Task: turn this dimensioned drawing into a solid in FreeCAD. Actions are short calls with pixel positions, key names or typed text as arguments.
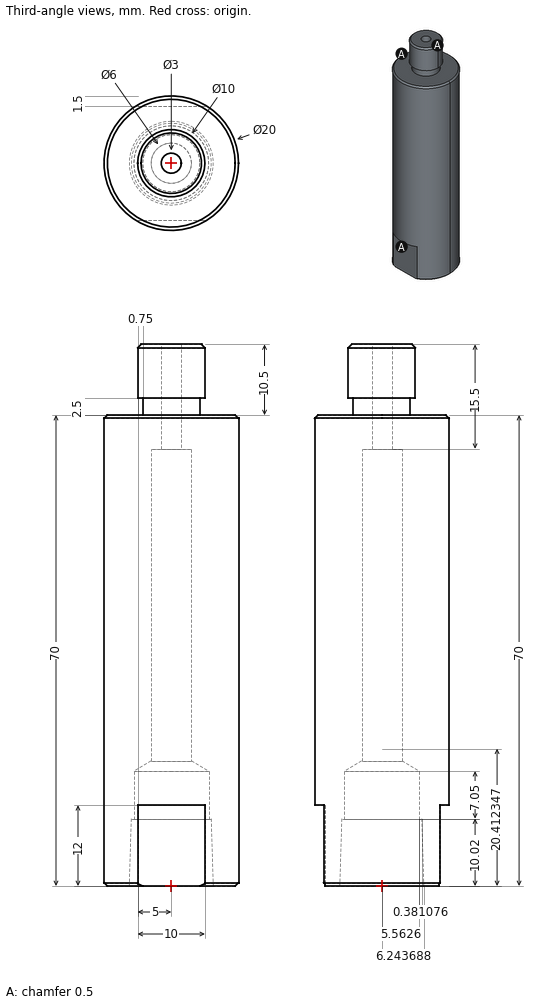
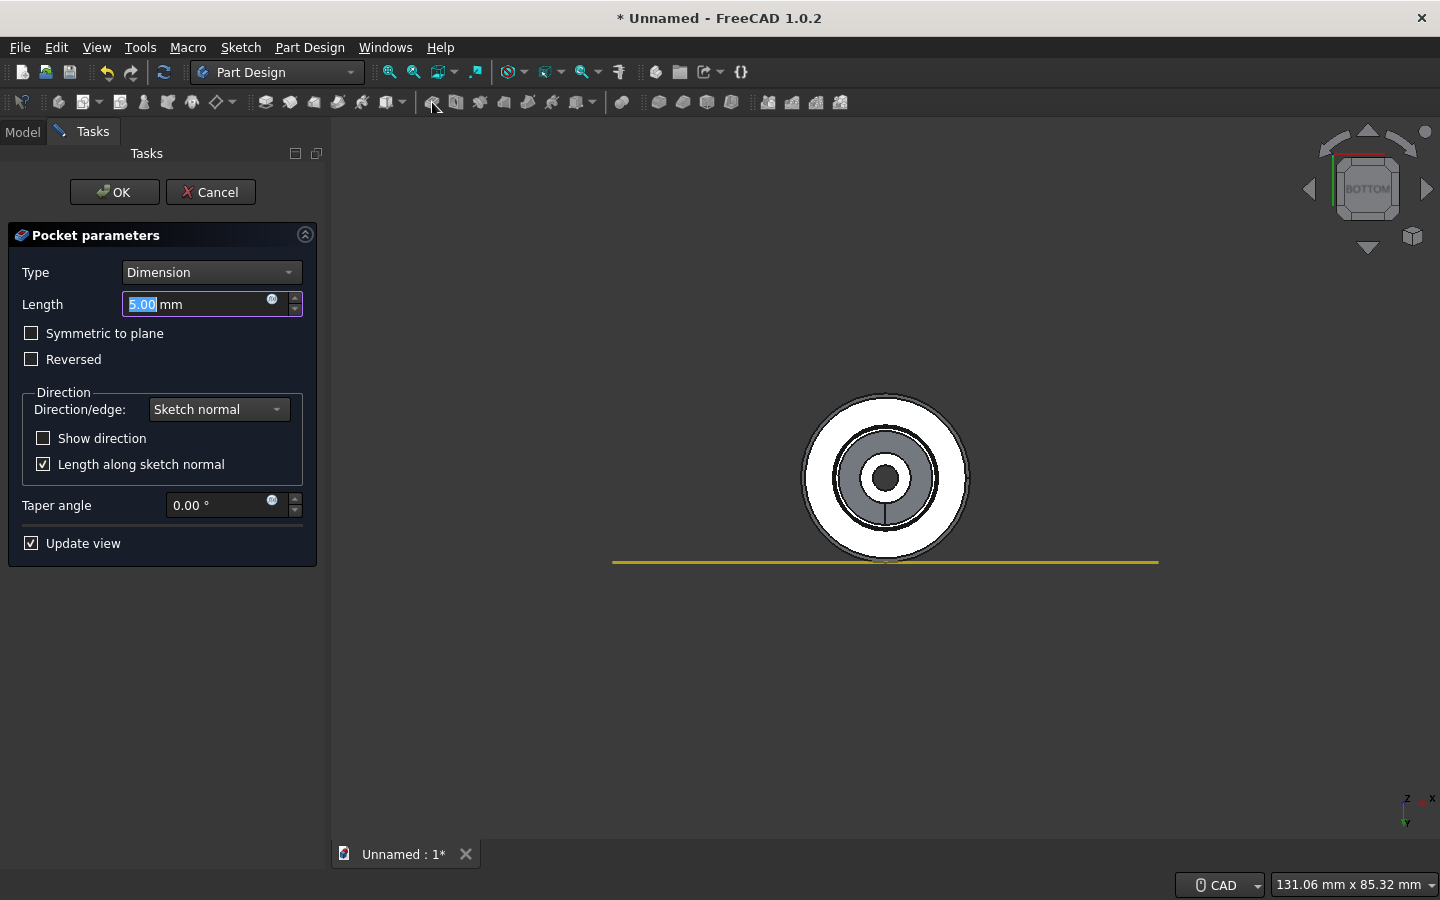
text(1.5)
key(Tab)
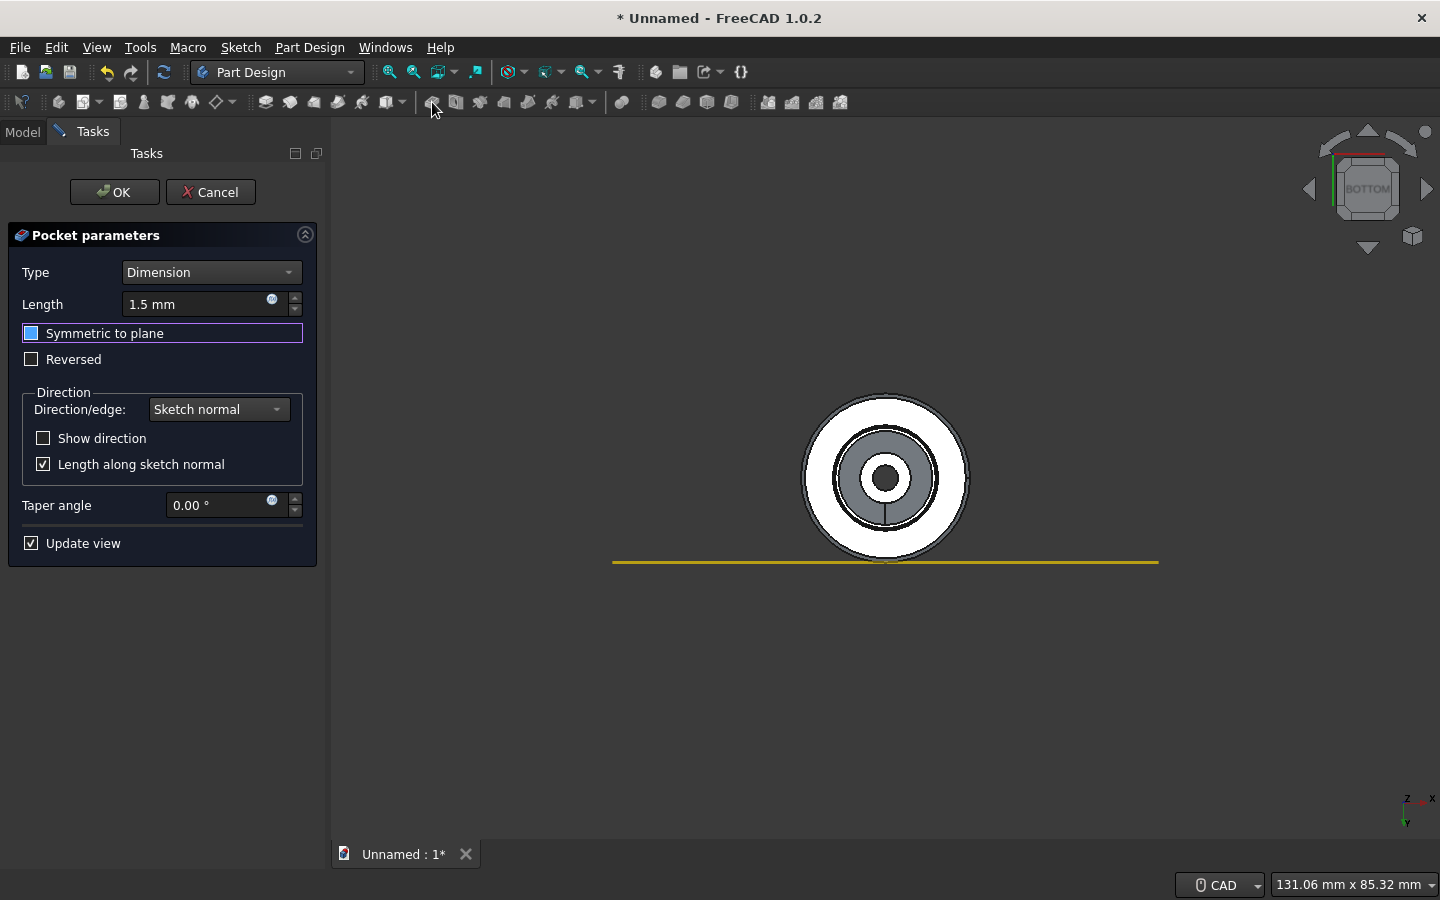
click(30, 359)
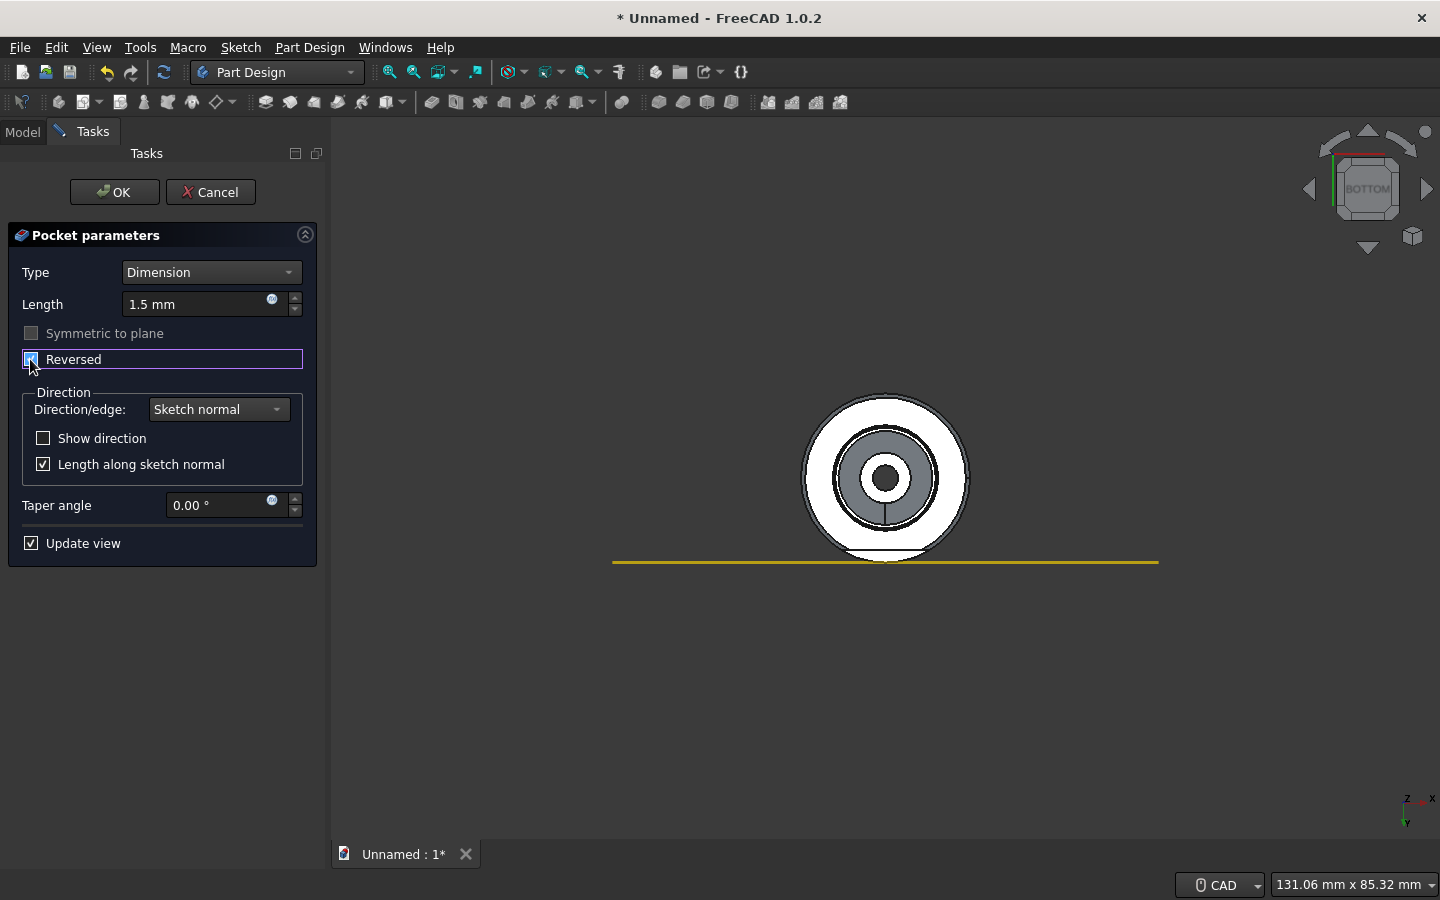
click(115, 192)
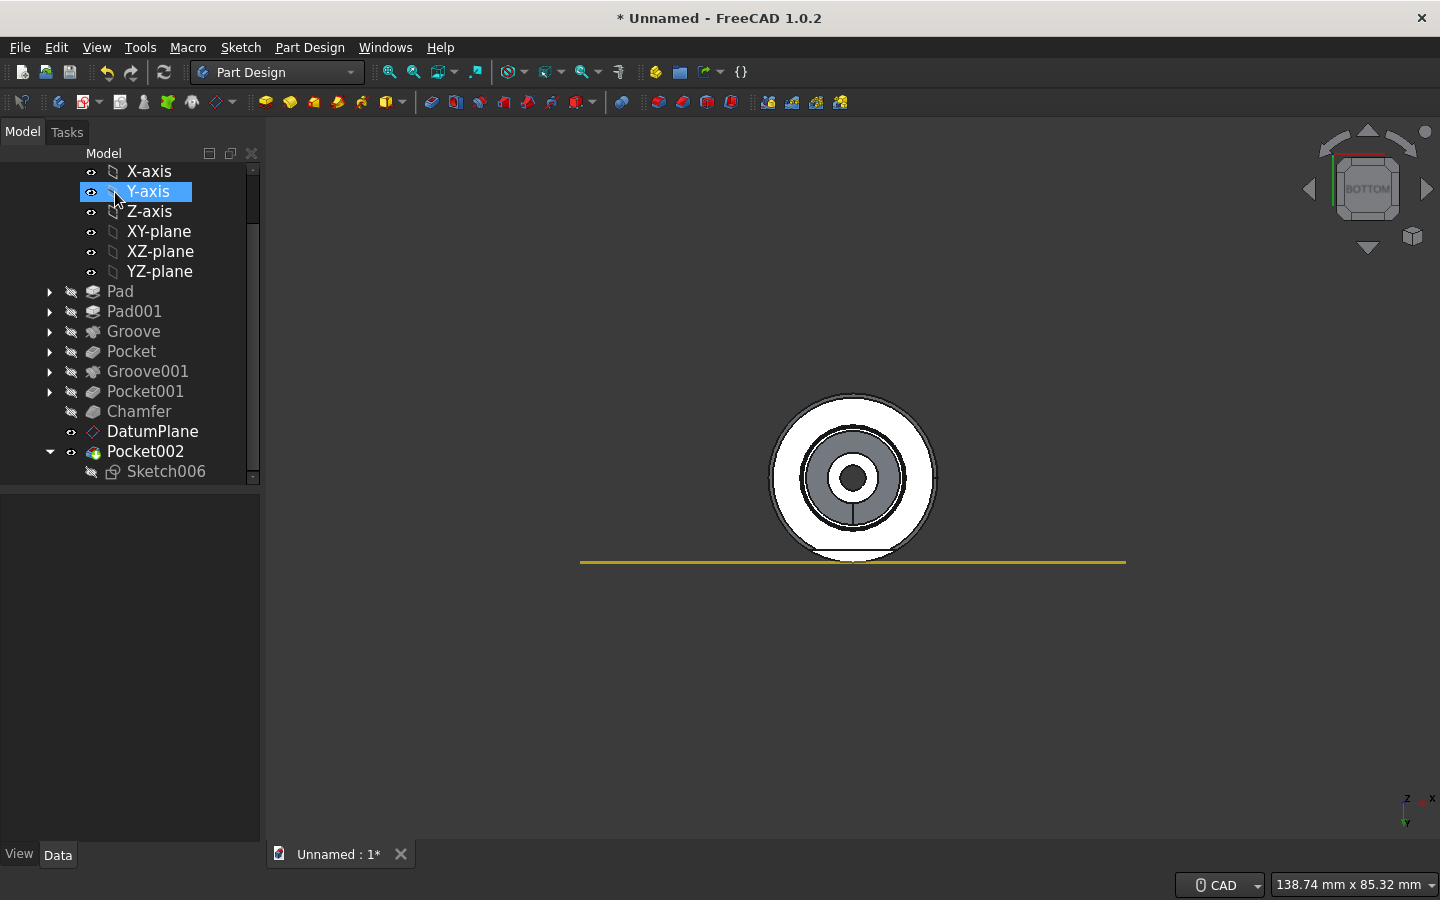
click(116, 432)
key(space)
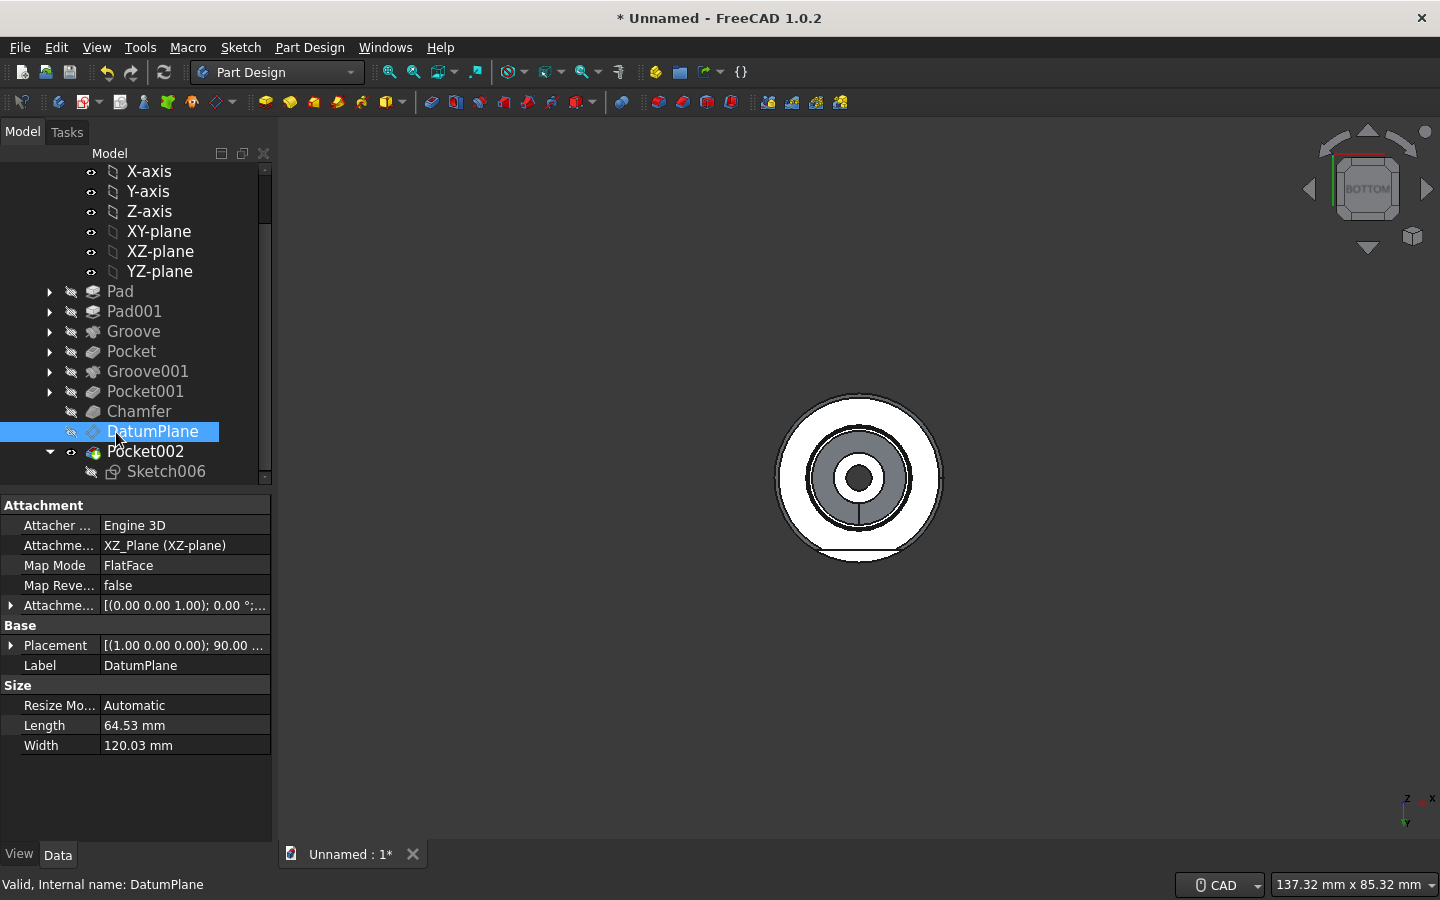
click(390, 72)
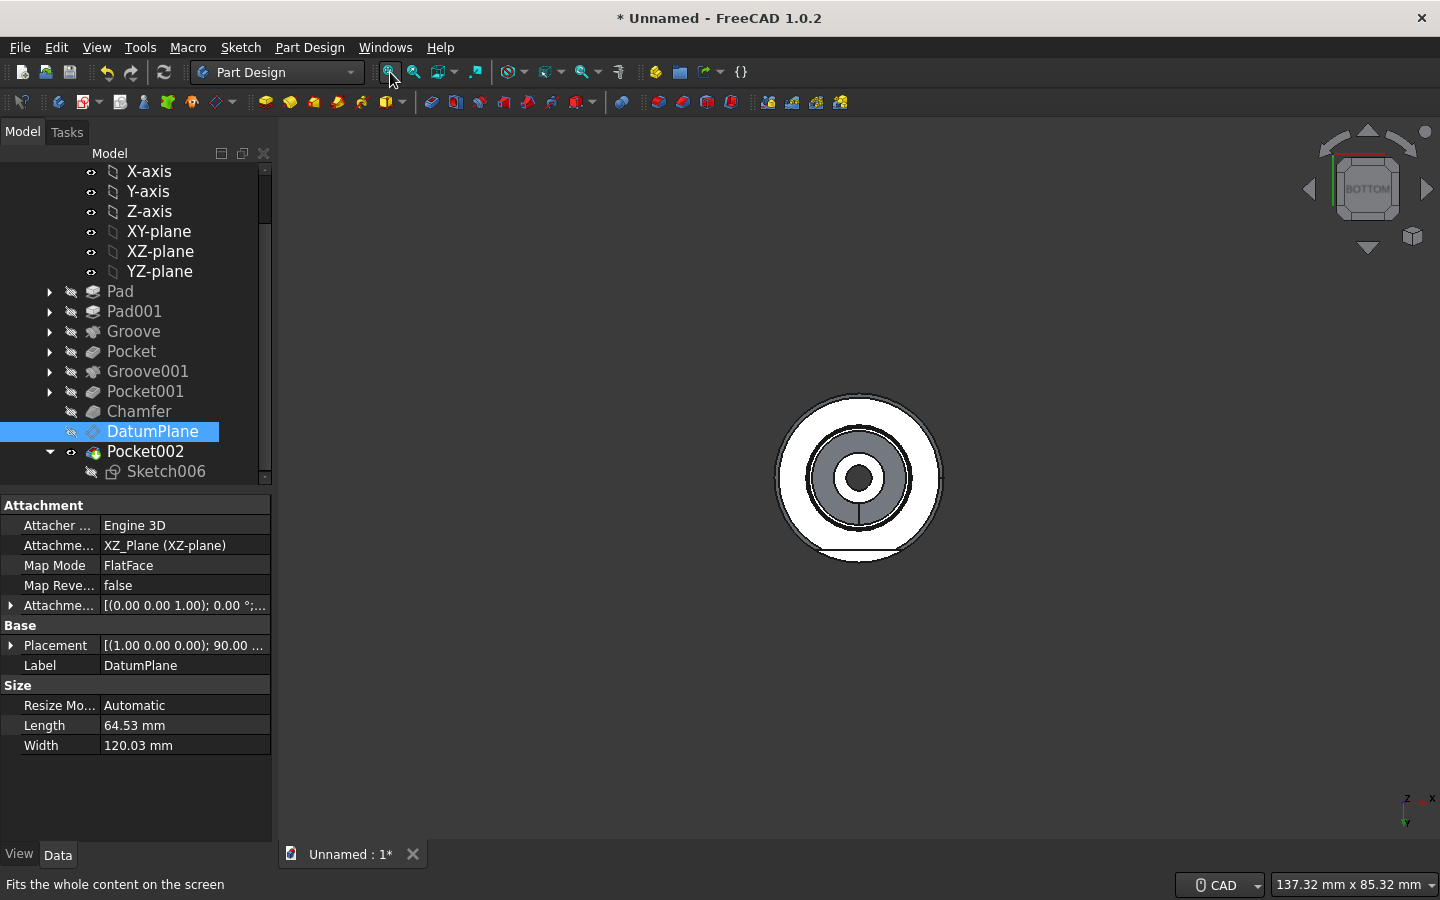
click(116, 452)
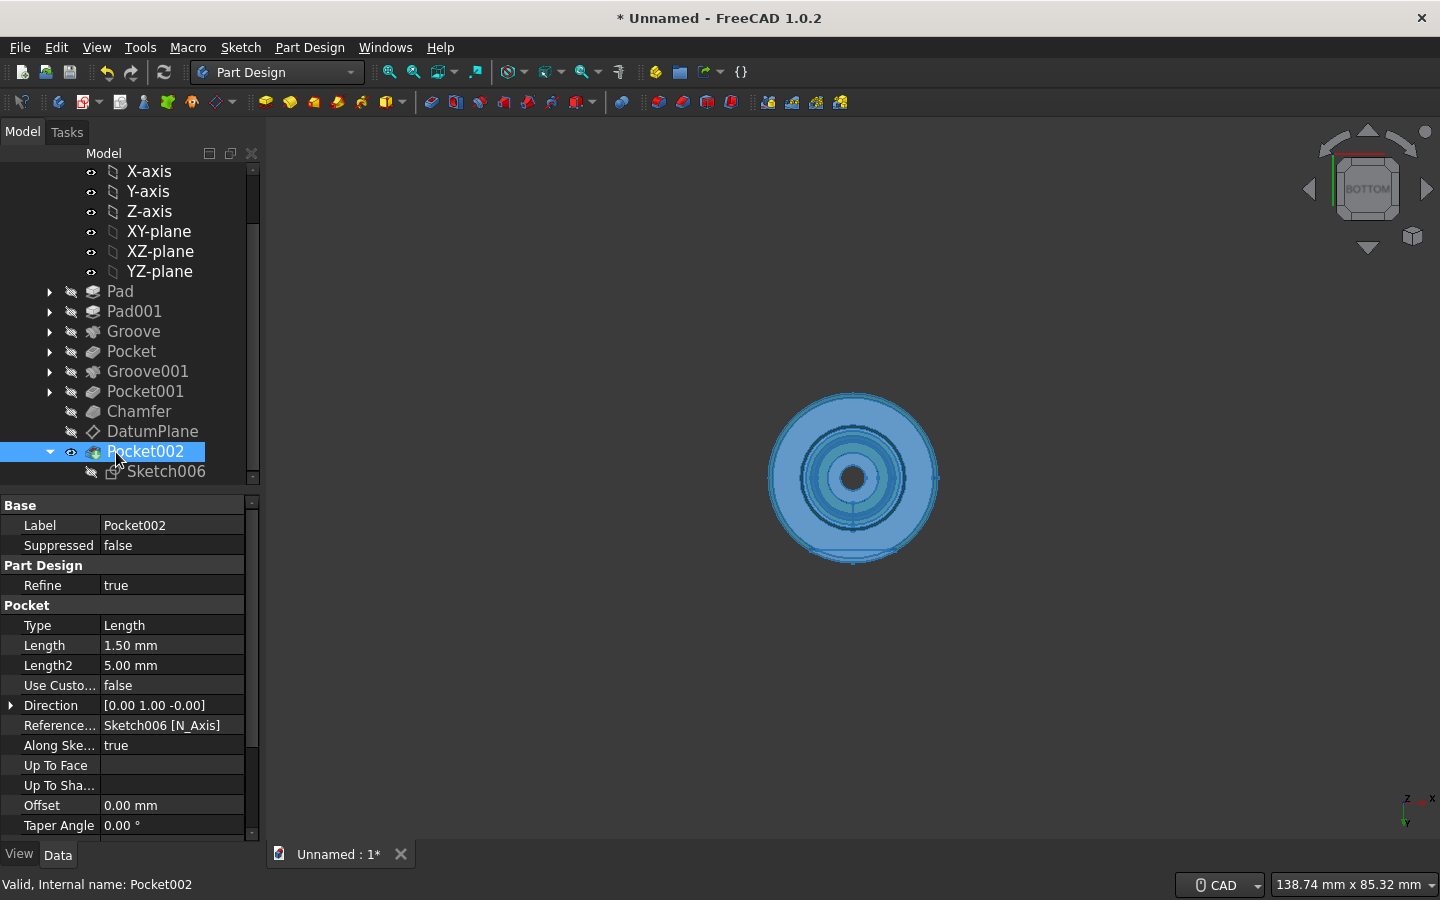
click(768, 102)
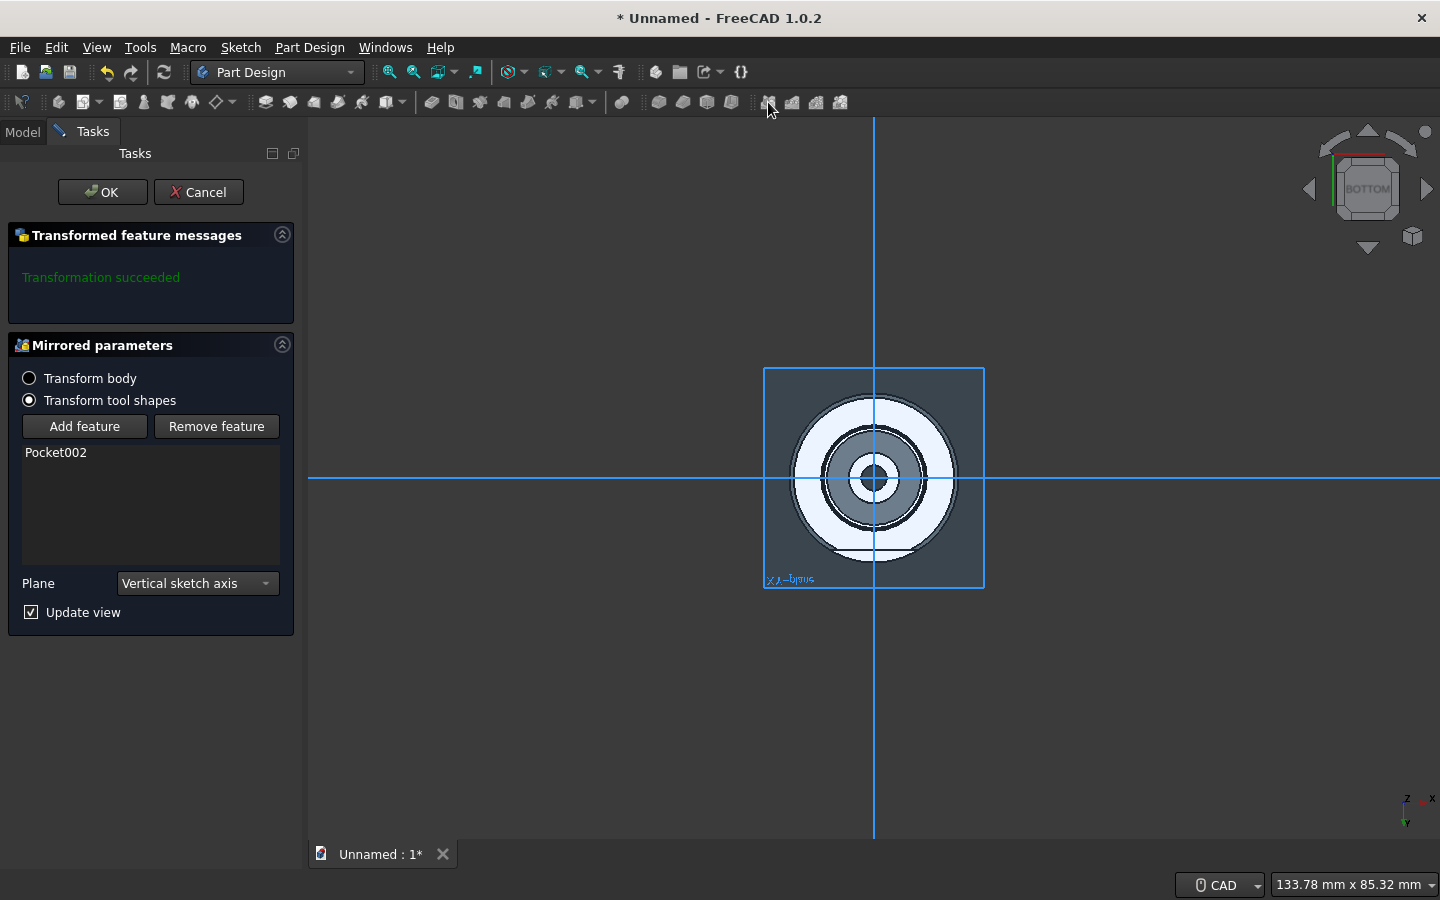
click(198, 584)